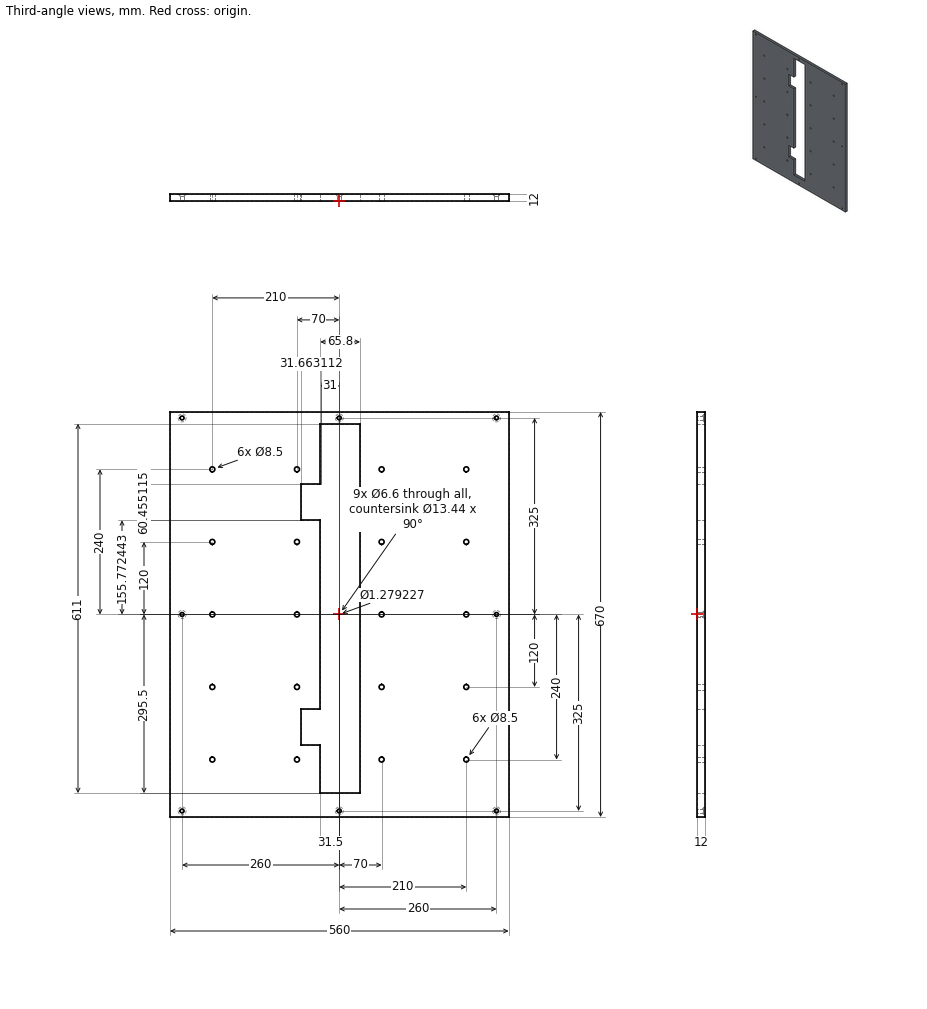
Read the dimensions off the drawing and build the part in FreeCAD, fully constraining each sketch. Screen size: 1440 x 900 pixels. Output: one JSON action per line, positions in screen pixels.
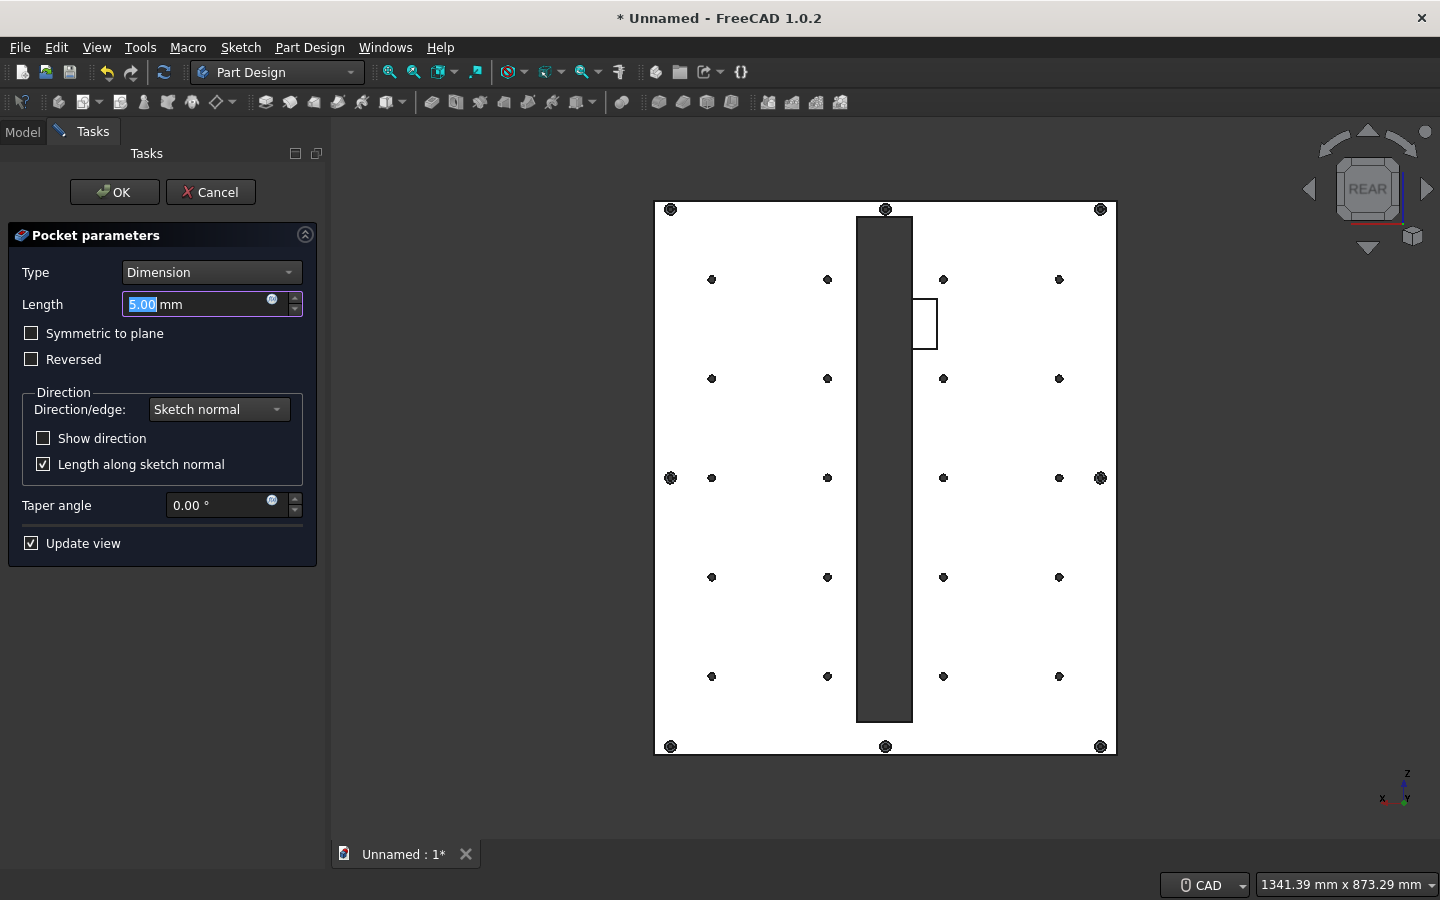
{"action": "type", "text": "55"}
{"action": "key", "text": "Tab"}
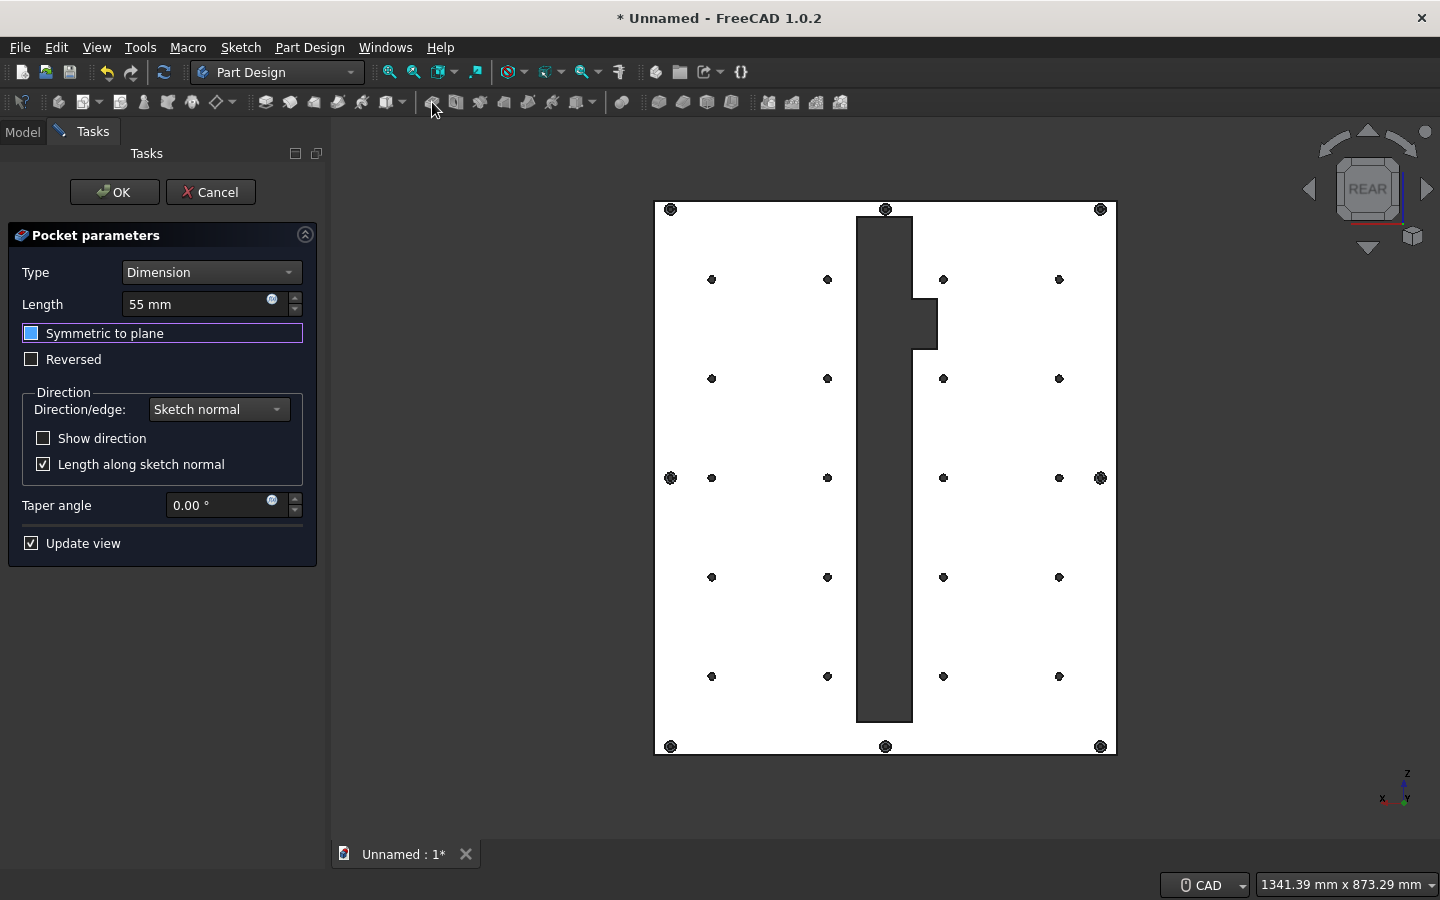
{"action": "left_click", "coordinate": [115, 192]}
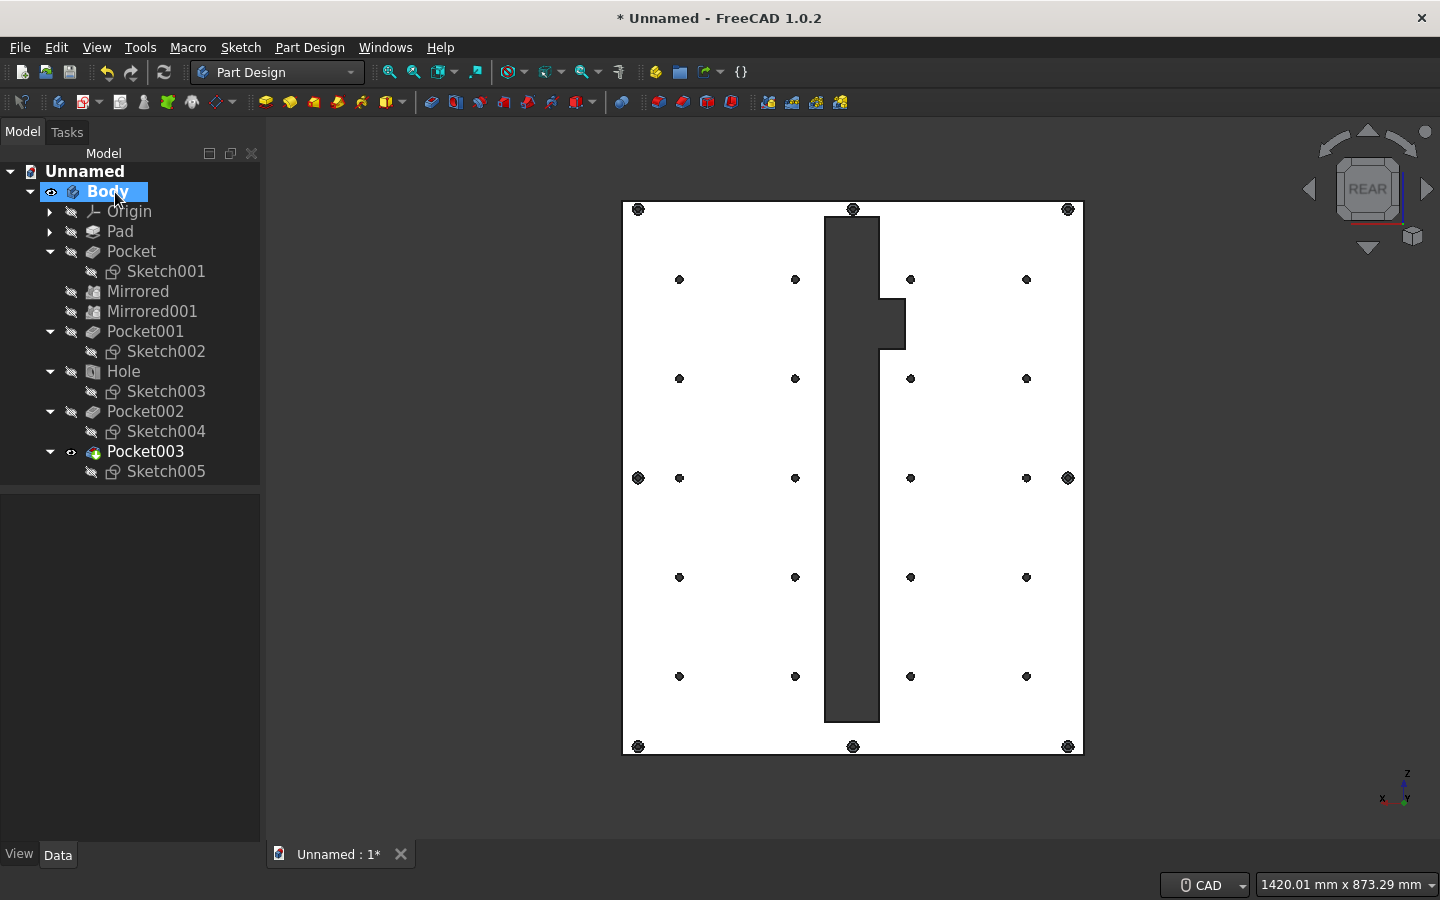
{"action": "left_click", "coordinate": [116, 452]}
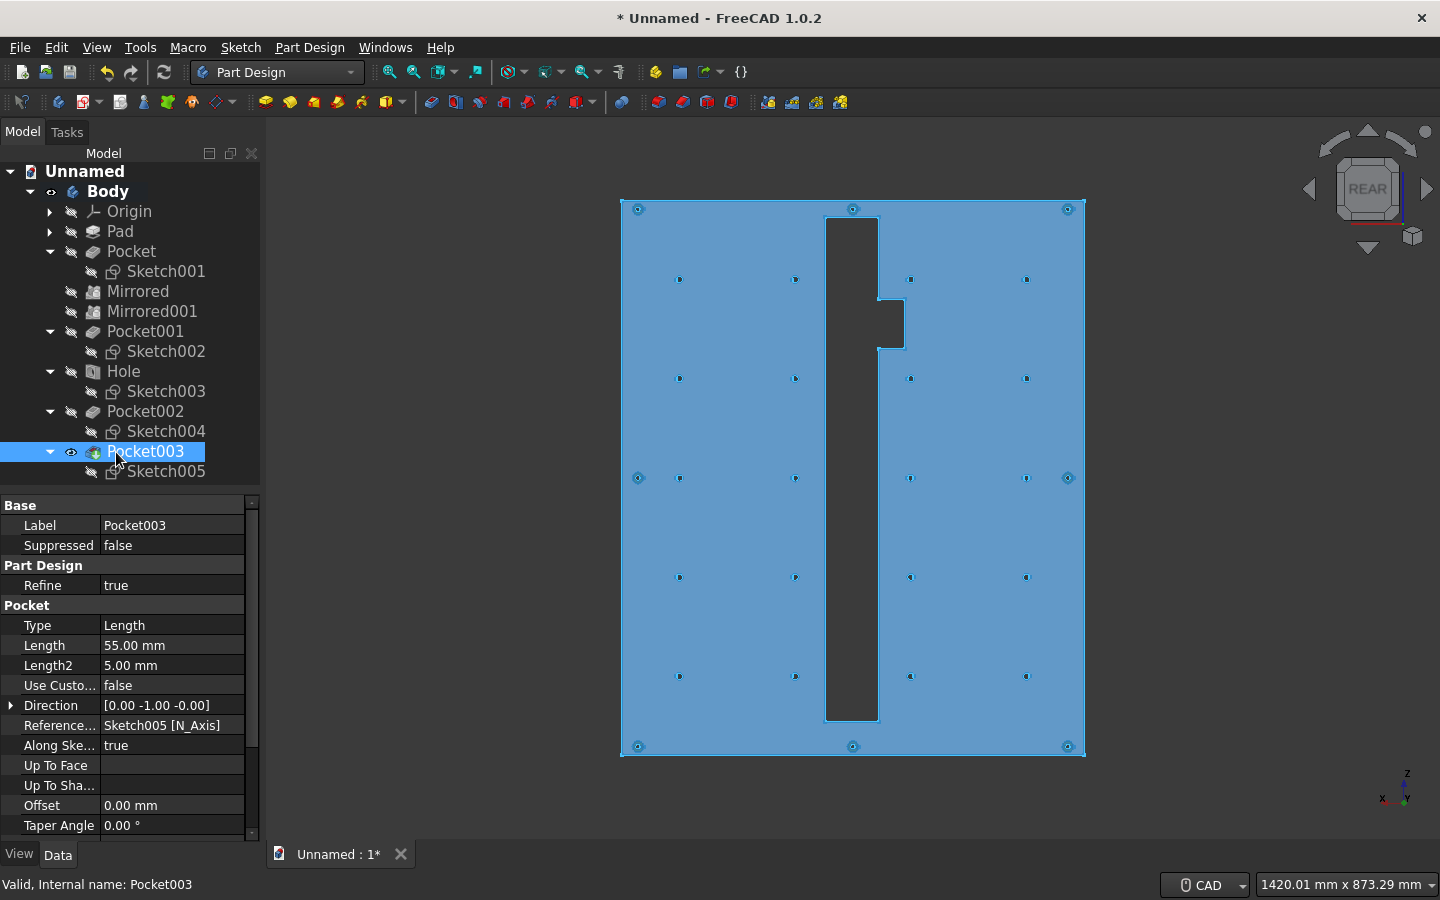
{"action": "left_click", "coordinate": [768, 102]}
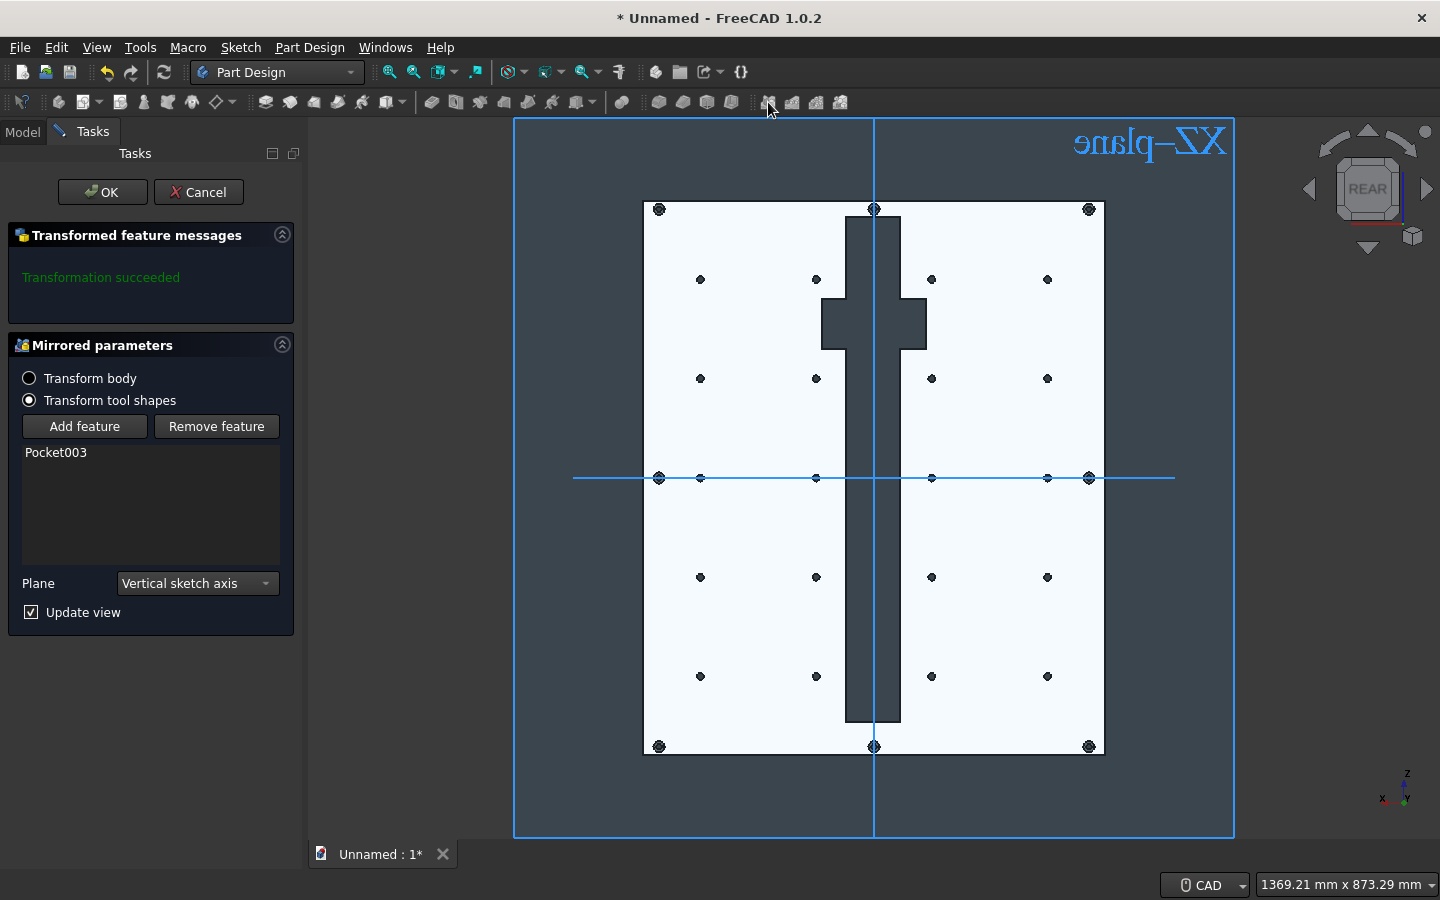
{"action": "left_click", "coordinate": [198, 584]}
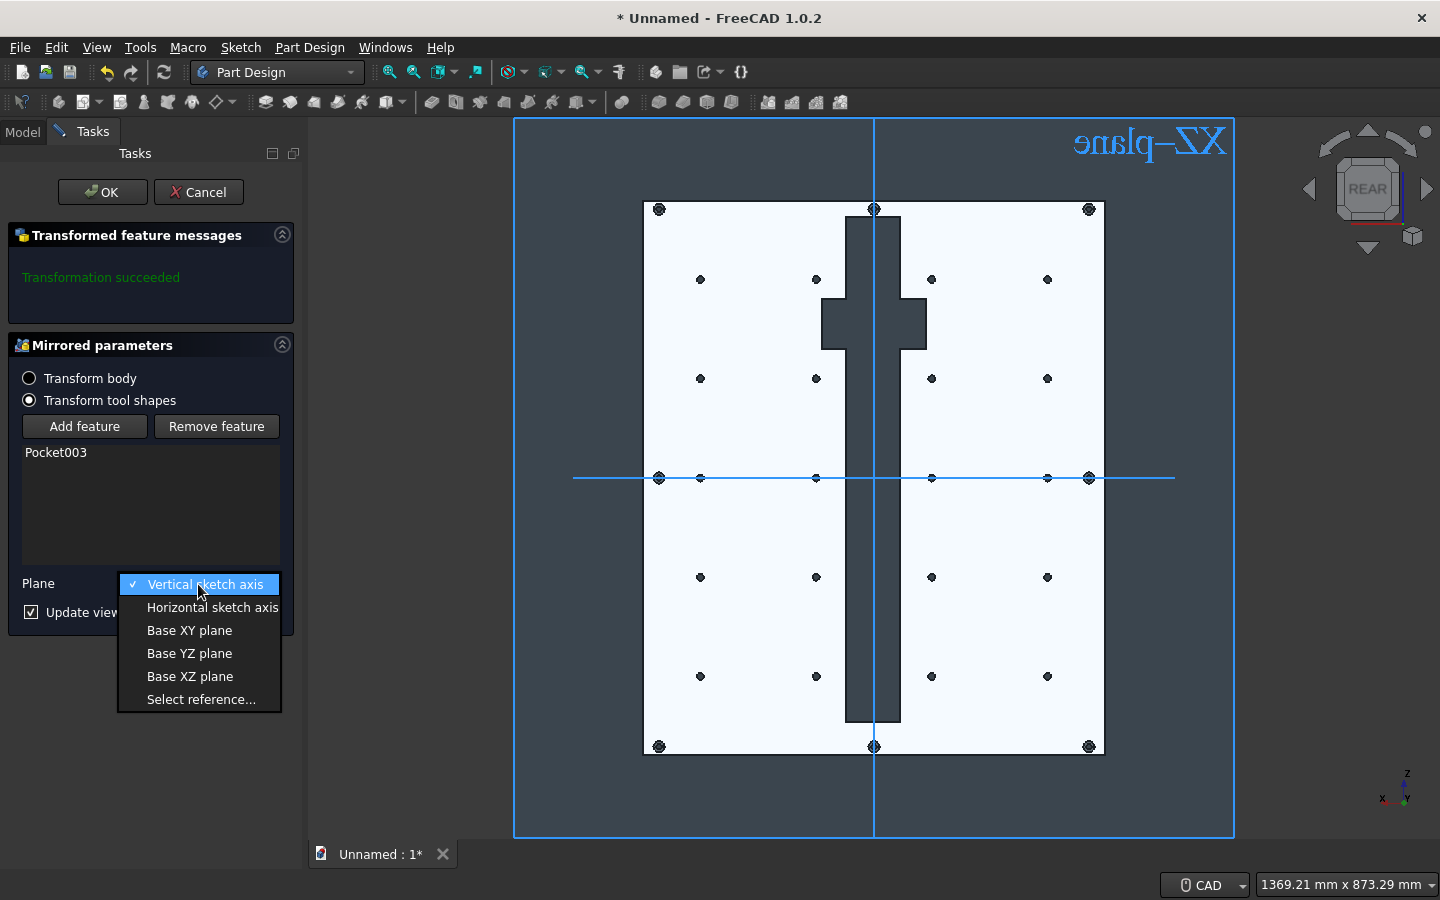
{"action": "left_click", "coordinate": [198, 630]}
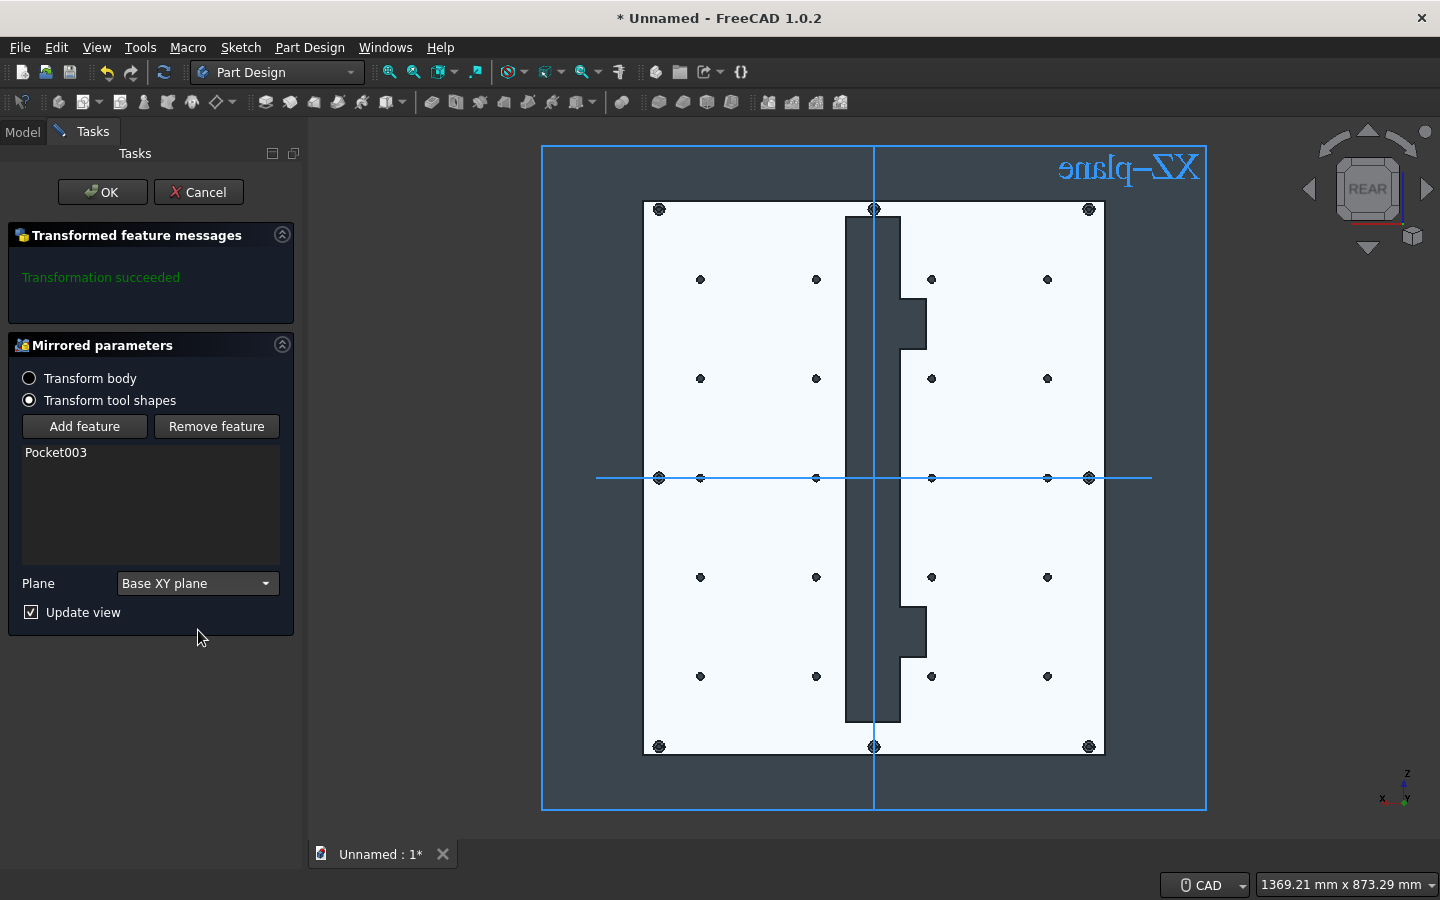
{"action": "left_click", "coordinate": [103, 192]}